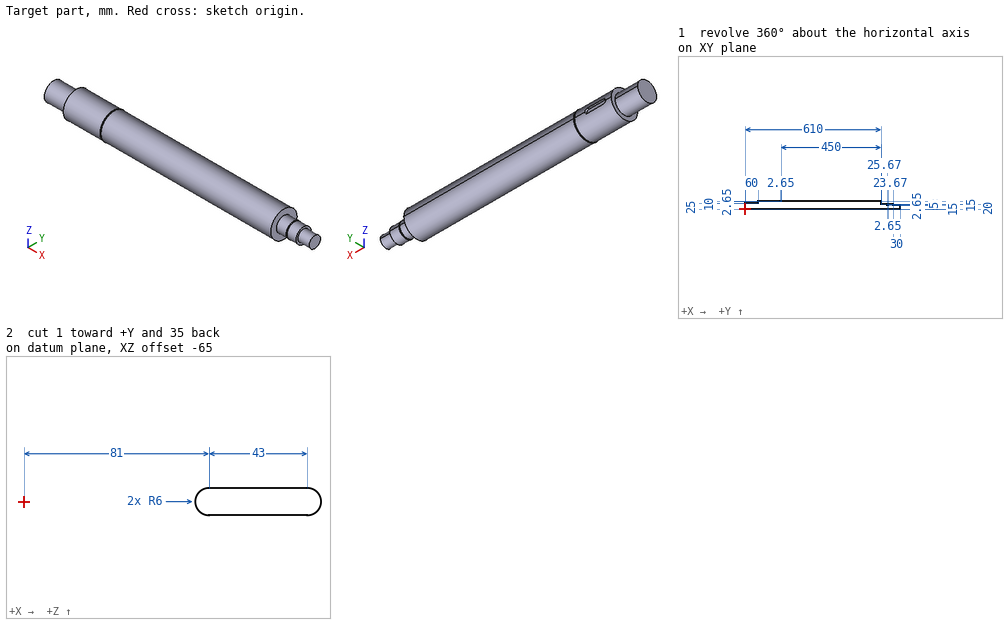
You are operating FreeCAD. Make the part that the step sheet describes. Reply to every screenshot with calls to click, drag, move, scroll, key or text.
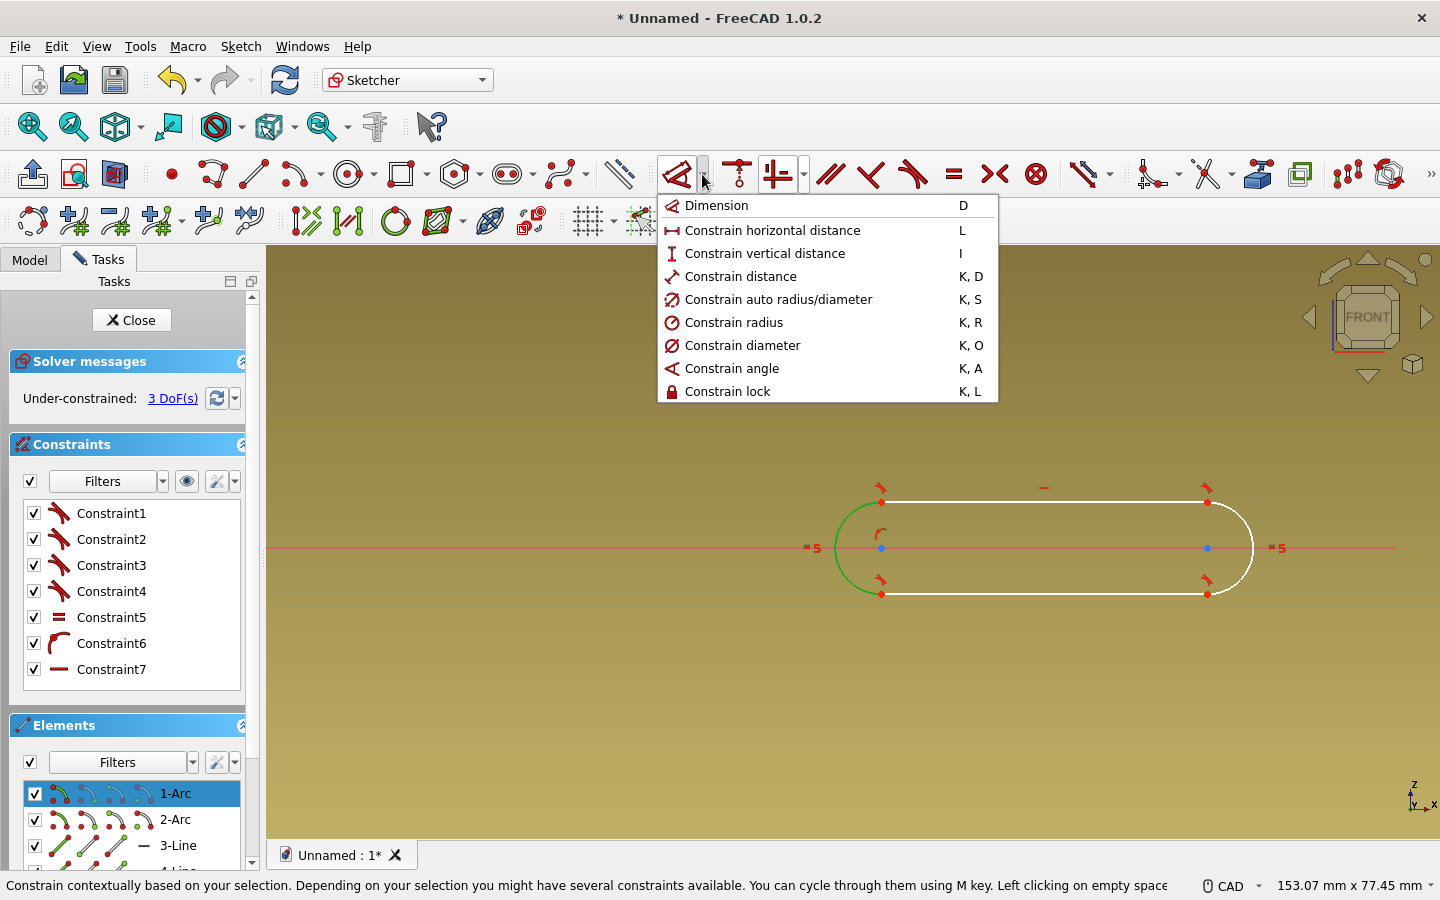
click(828, 322)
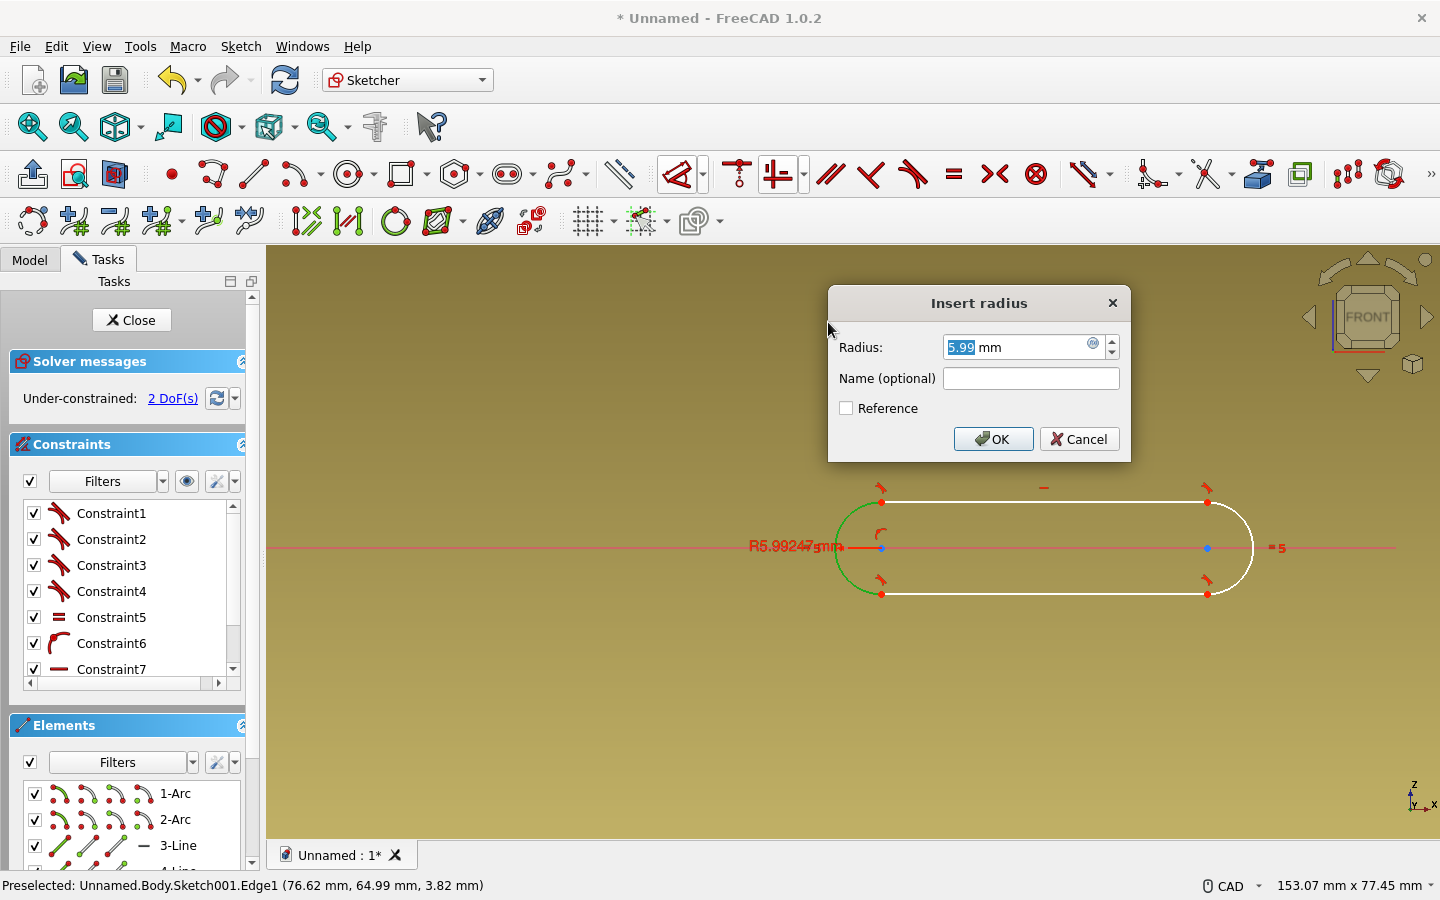
text(6)
key(Return)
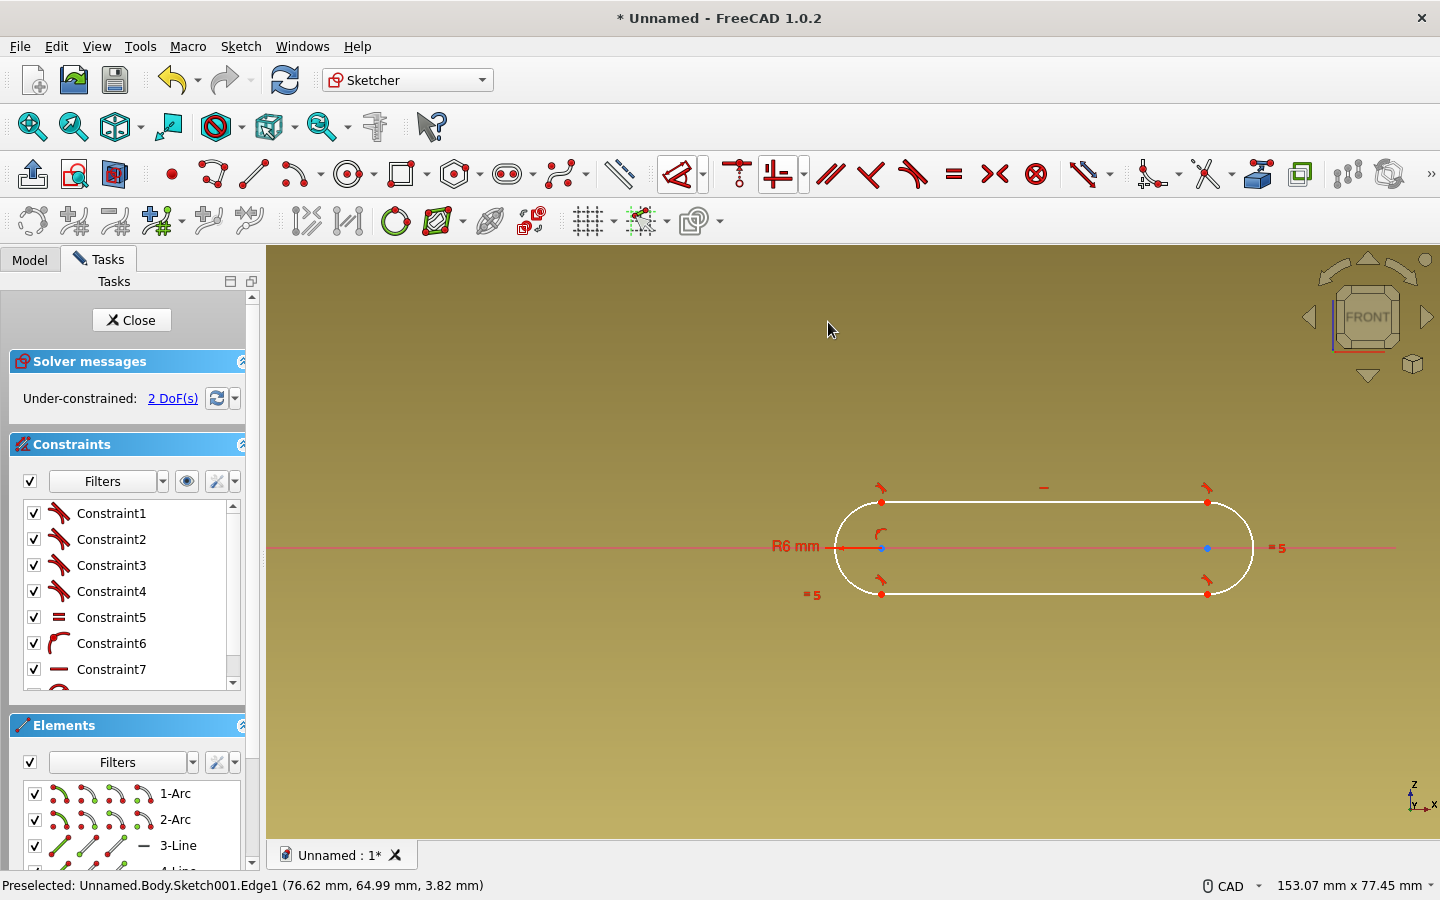
click(979, 502)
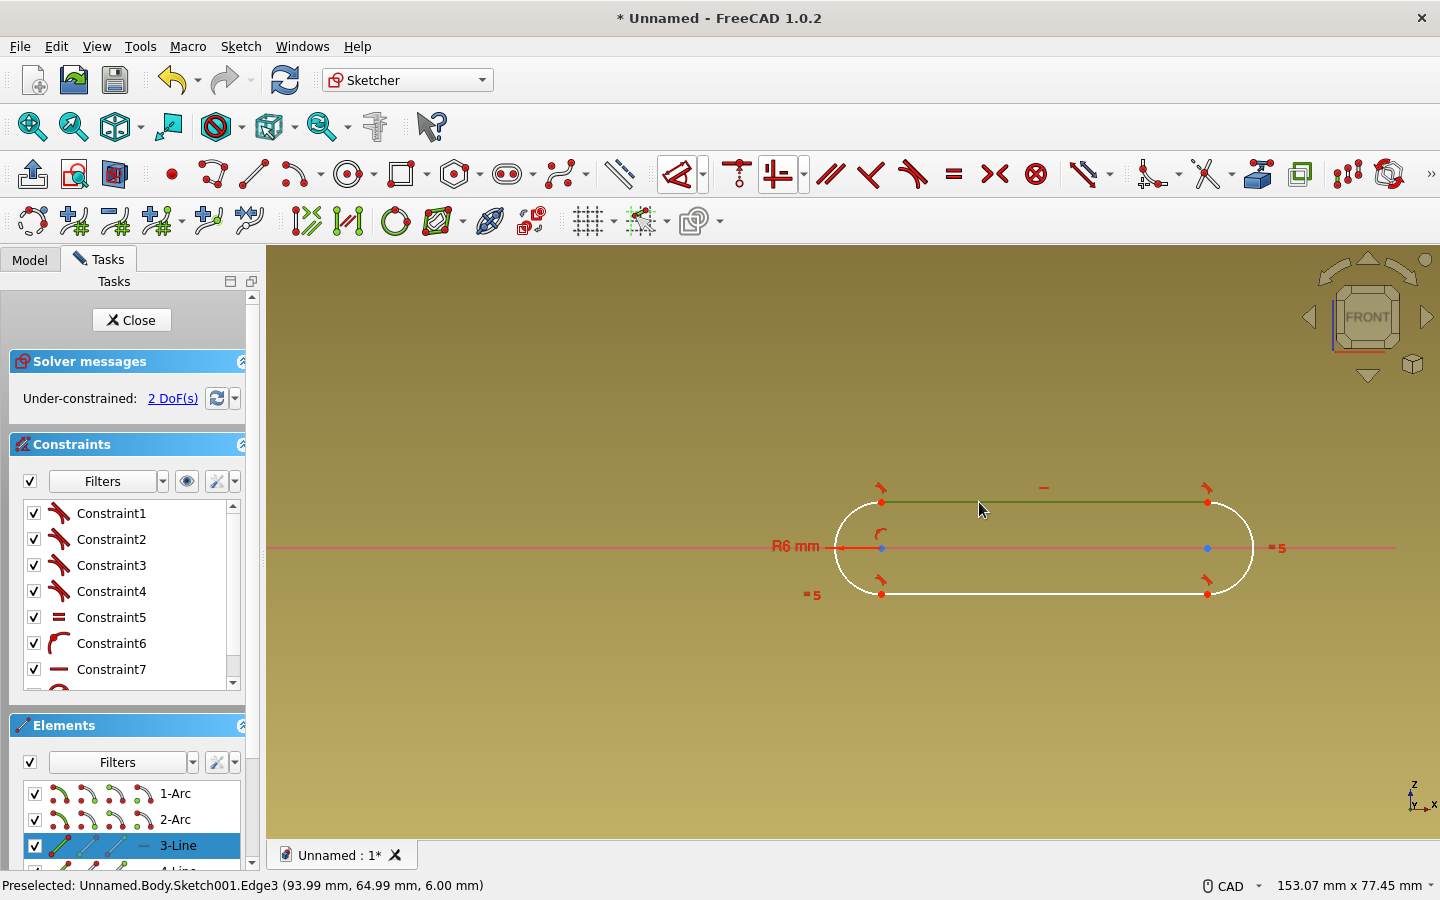
click(702, 174)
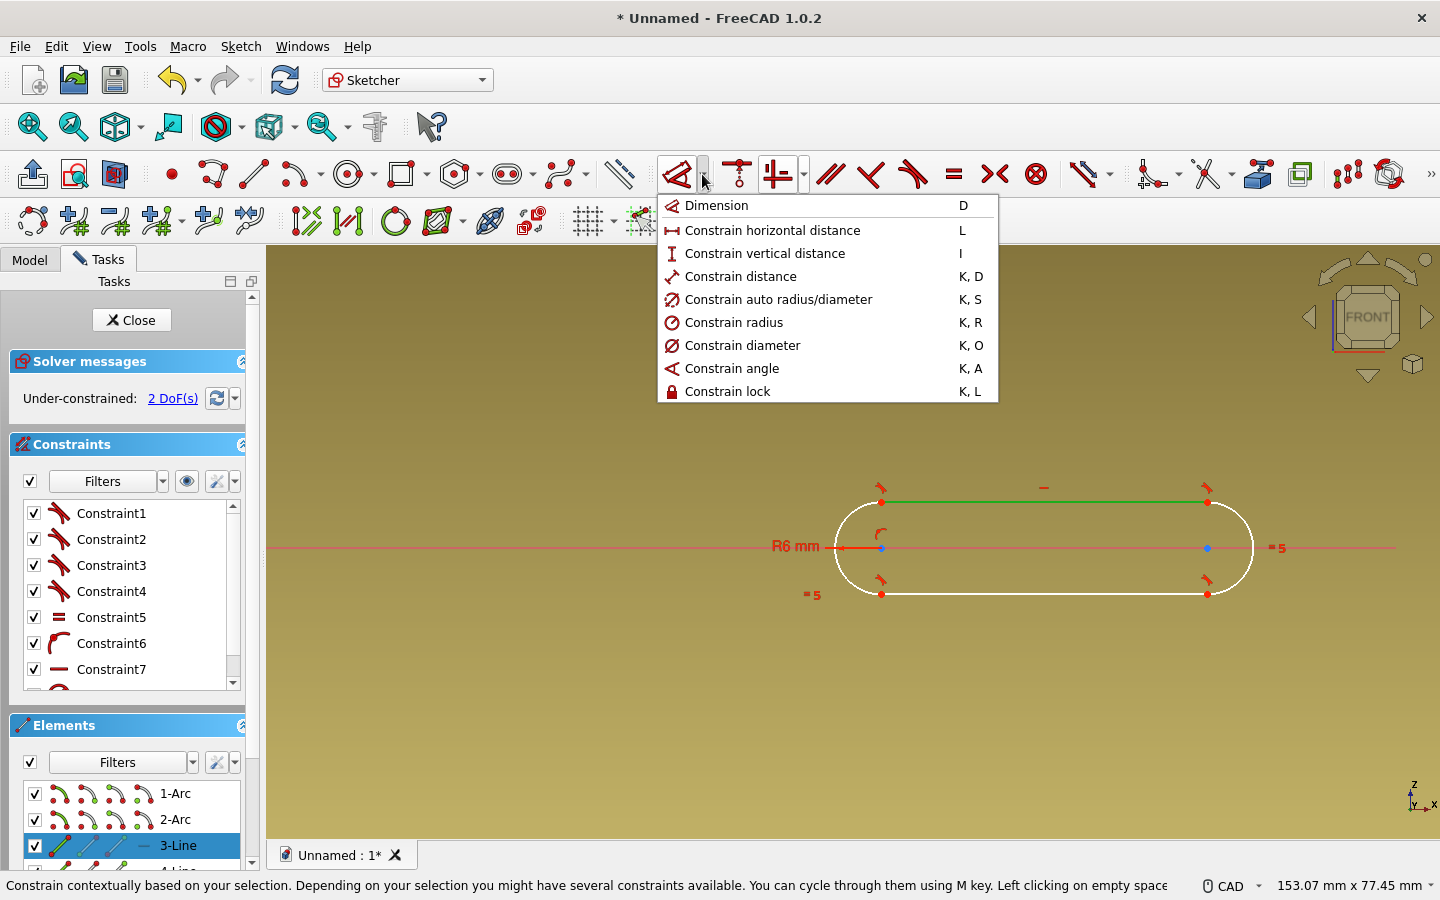
click(828, 230)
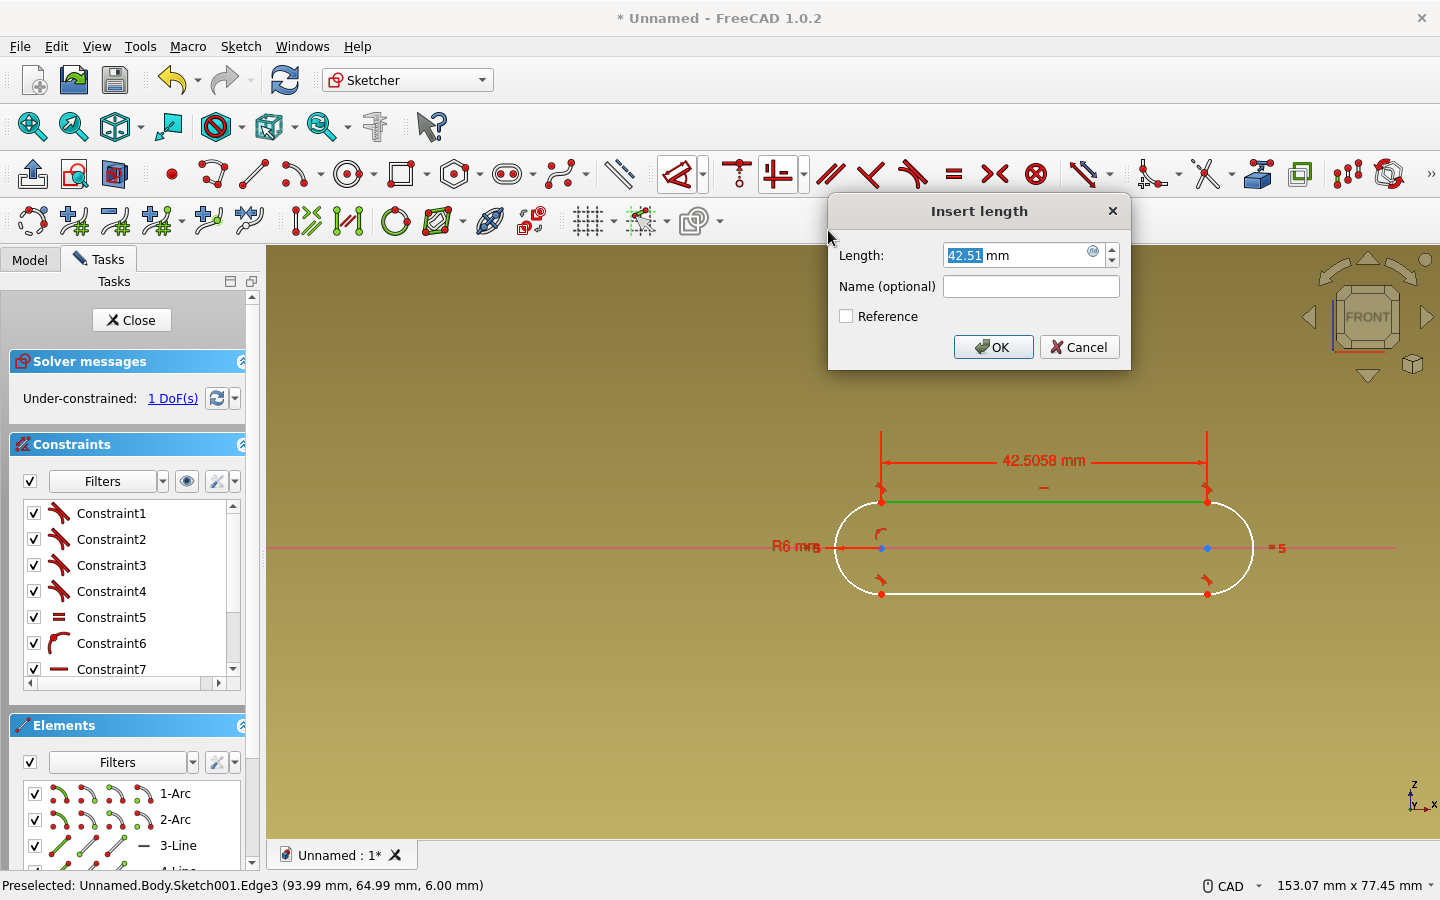
text(43)
key(Return)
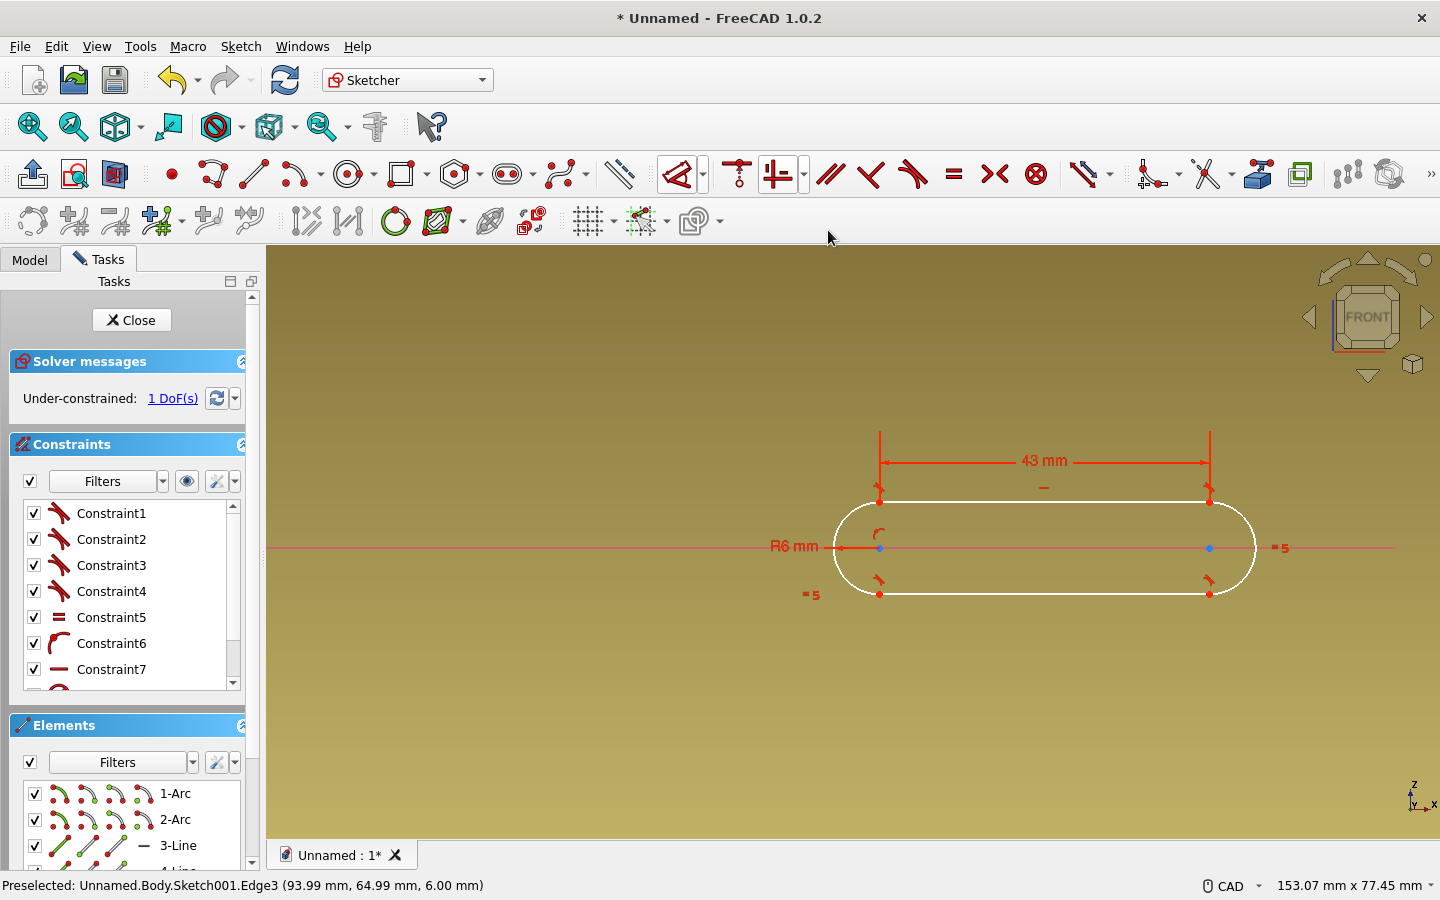
click(880, 502)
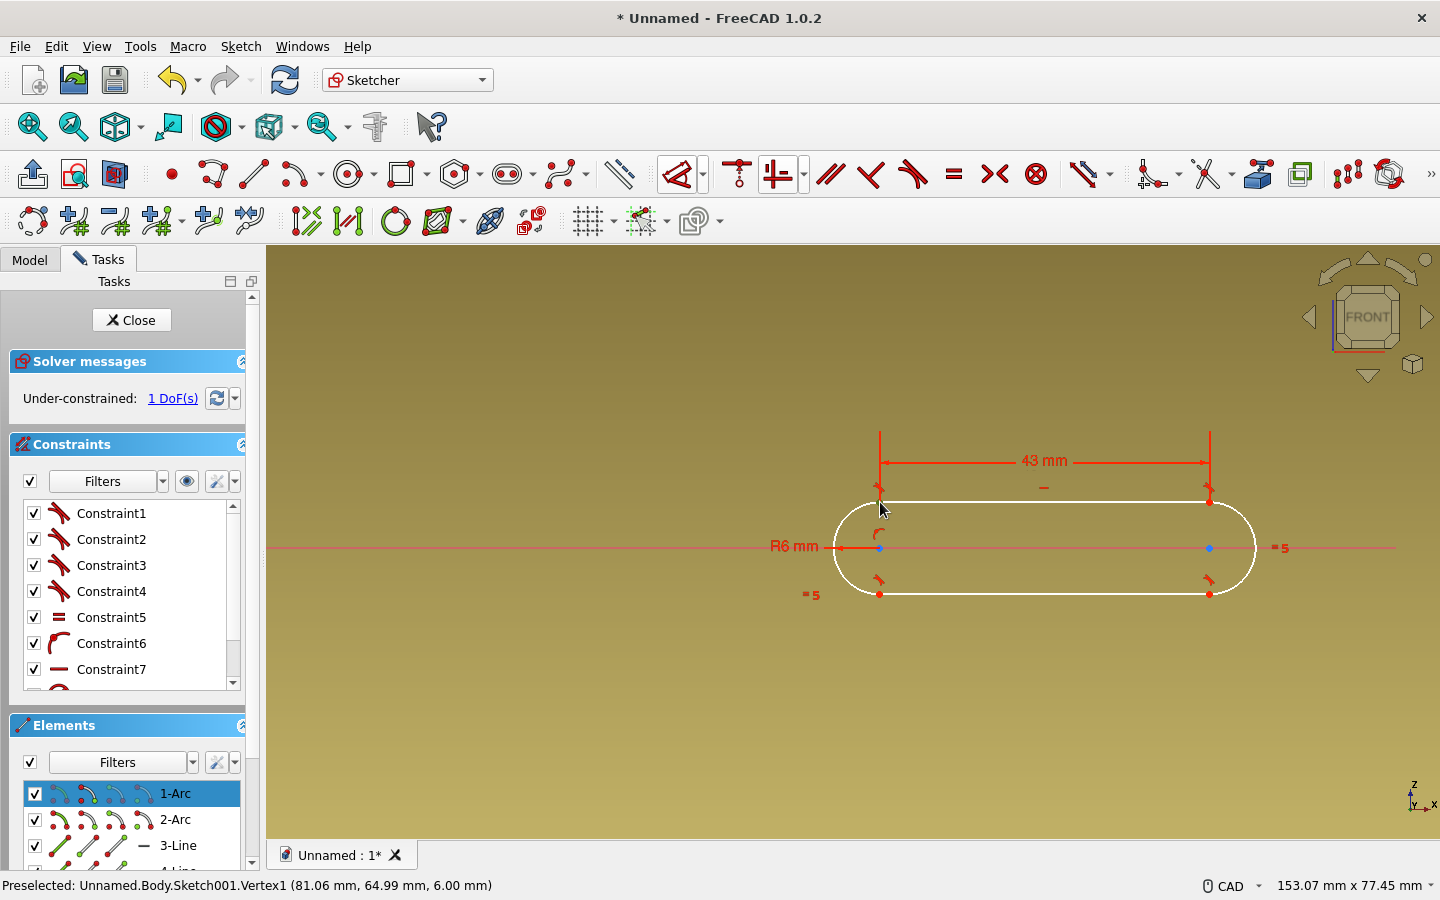
key(l)